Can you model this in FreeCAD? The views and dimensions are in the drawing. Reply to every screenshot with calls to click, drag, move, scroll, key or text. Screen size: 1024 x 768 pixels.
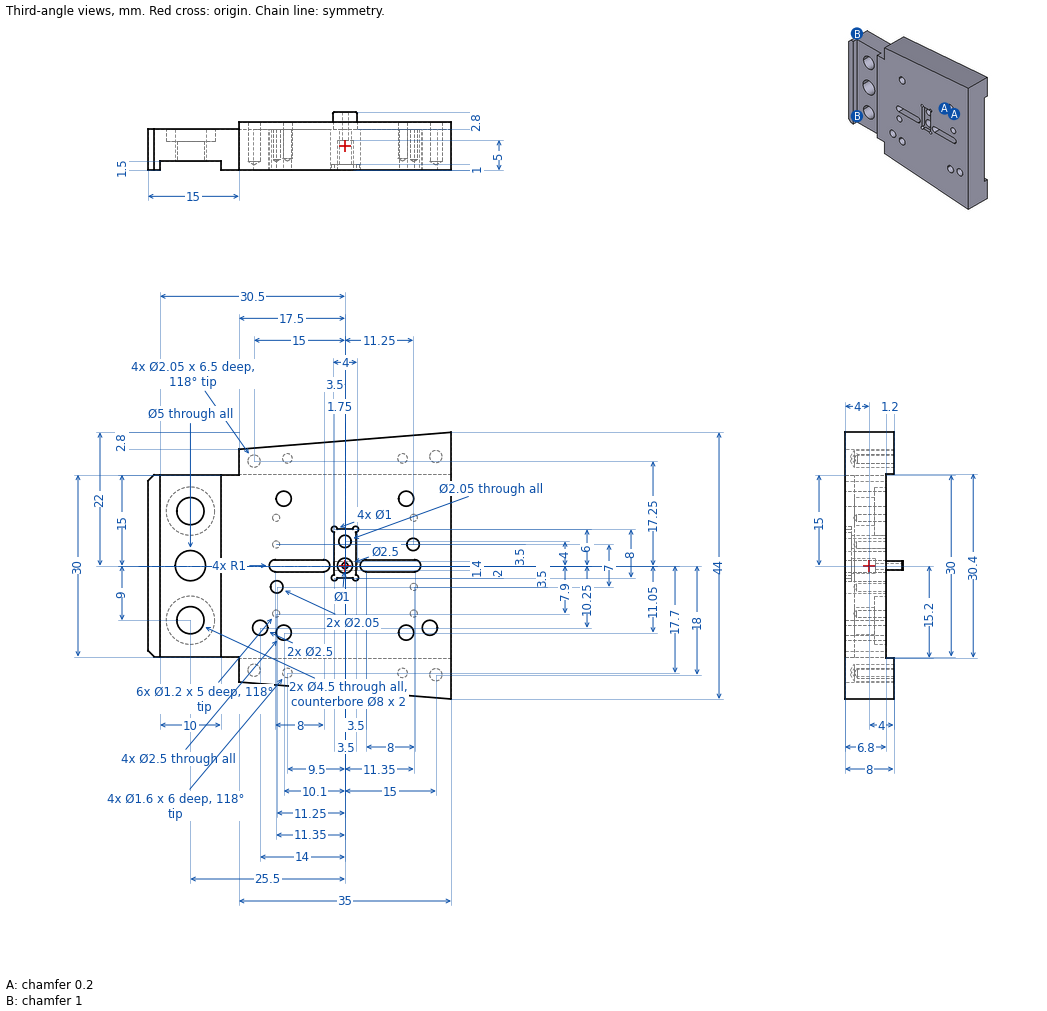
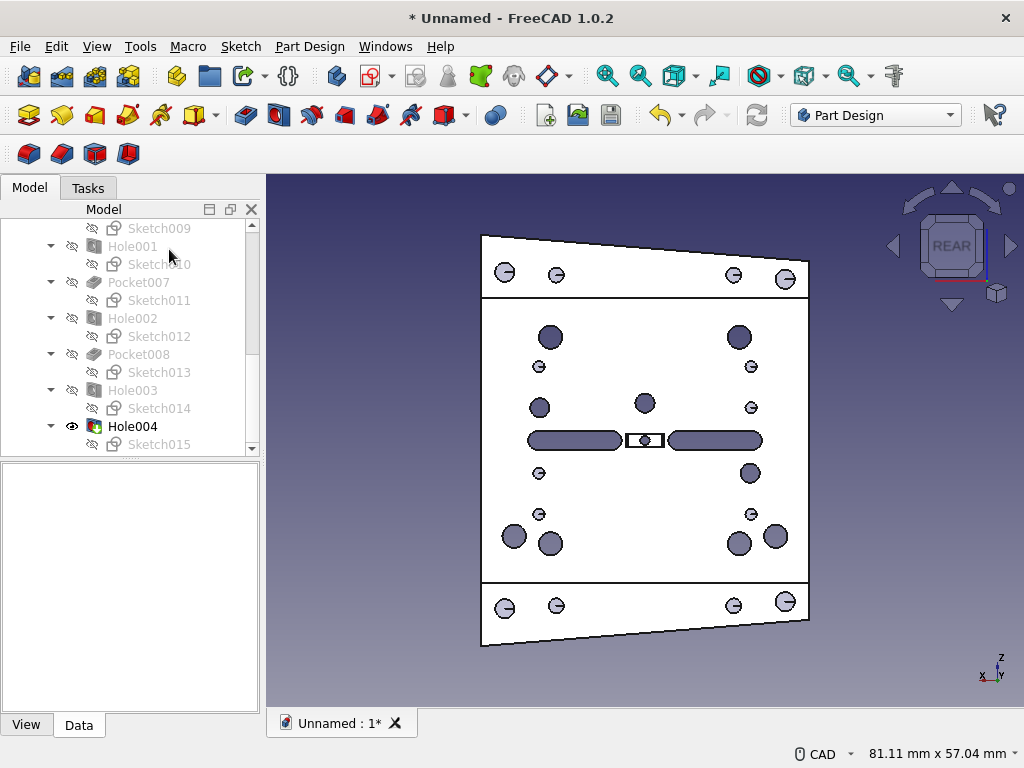
key(6)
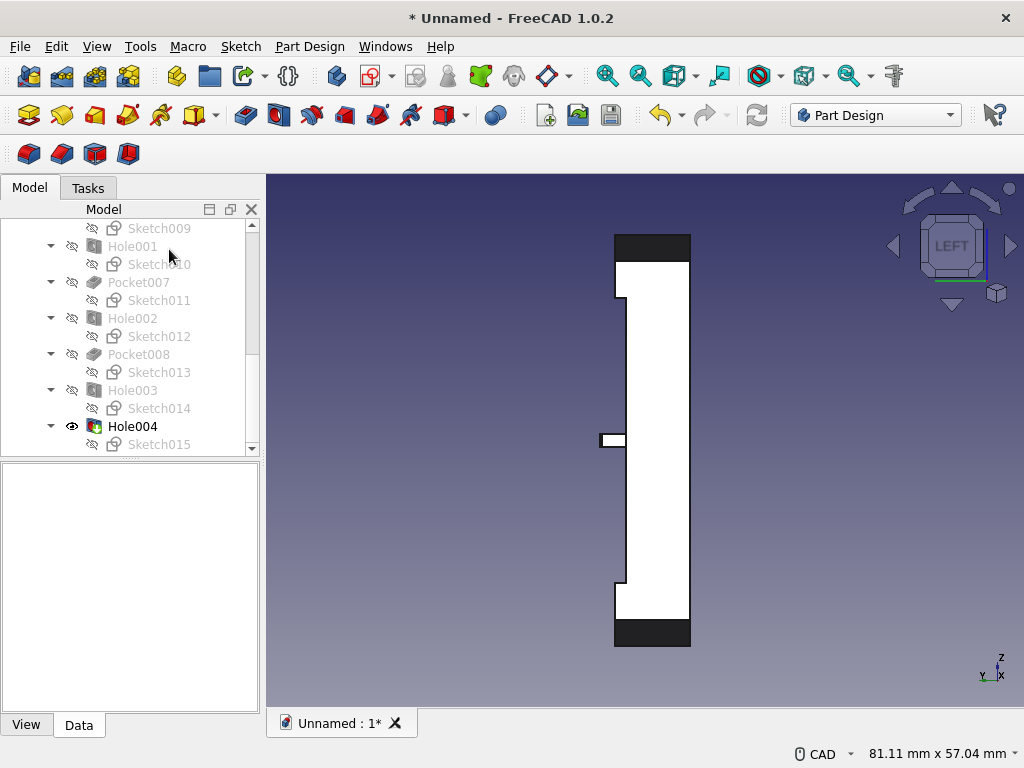
click(663, 440)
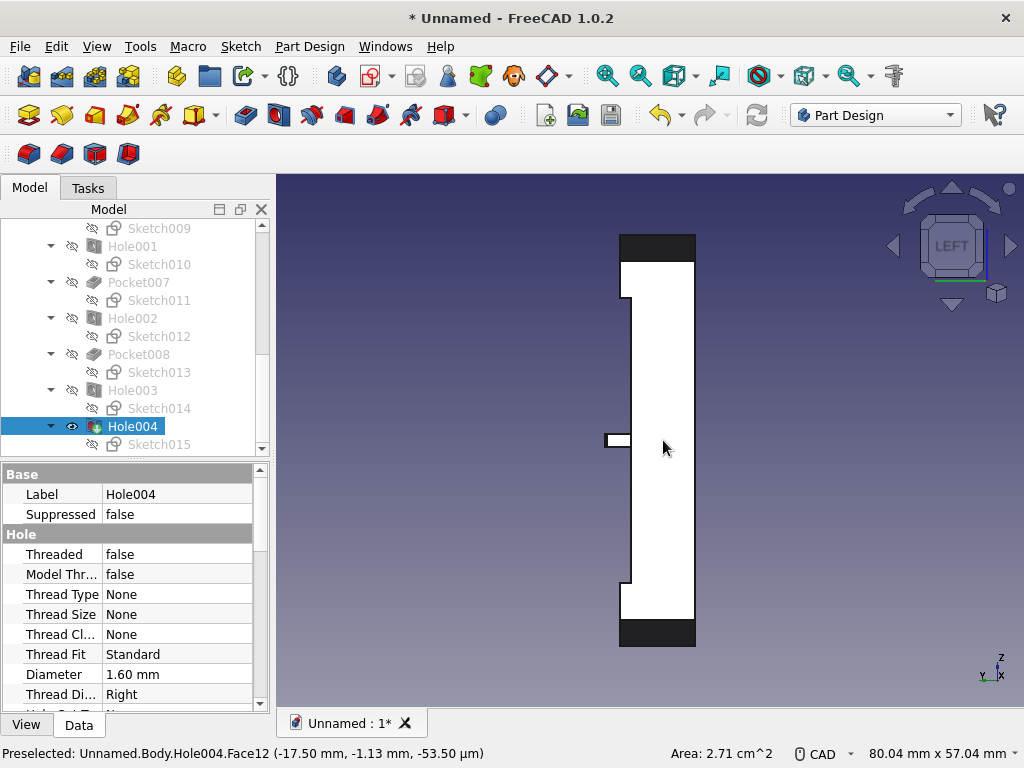
click(370, 76)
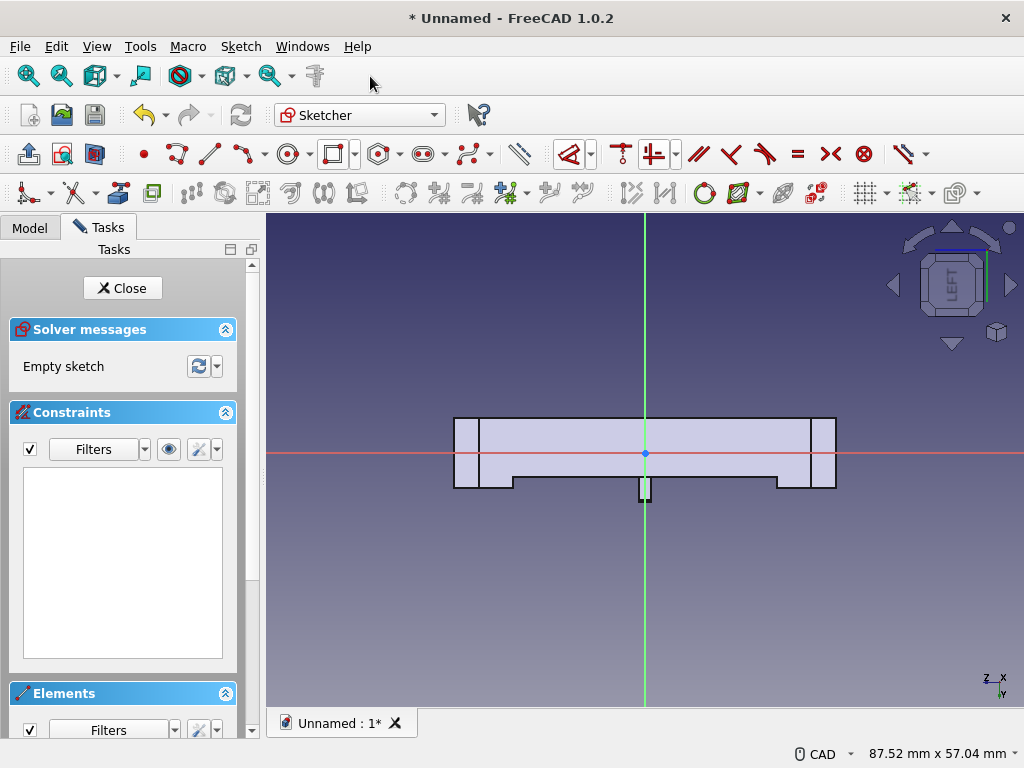
scroll(784, 423, up, 2)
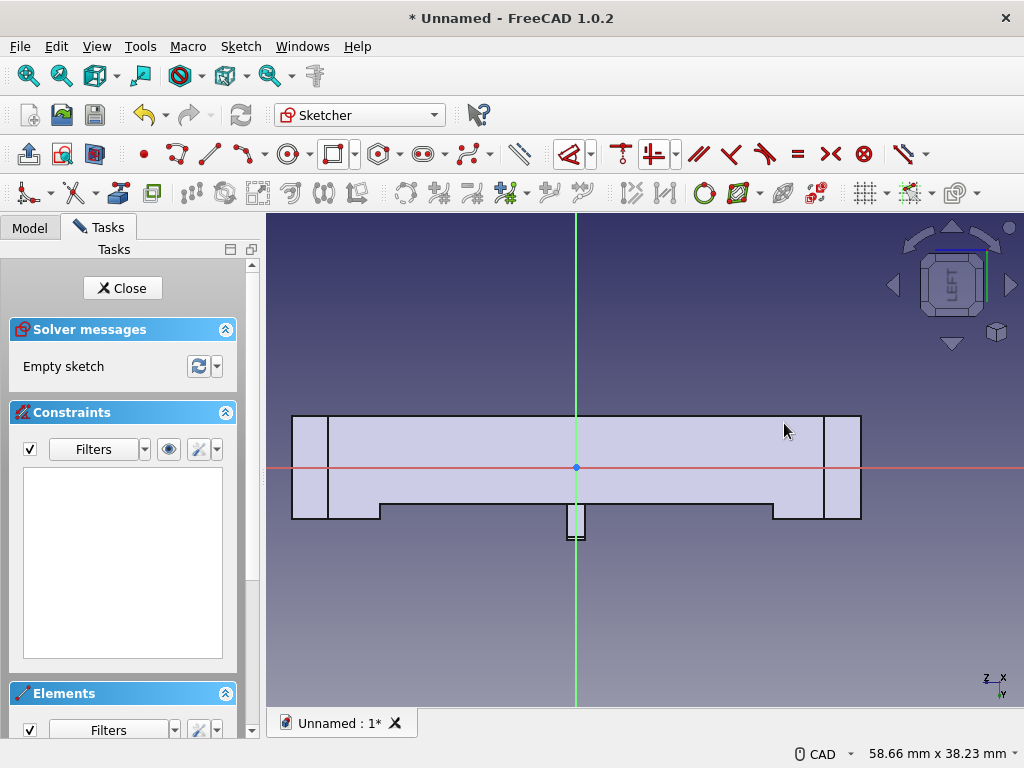
click(332, 154)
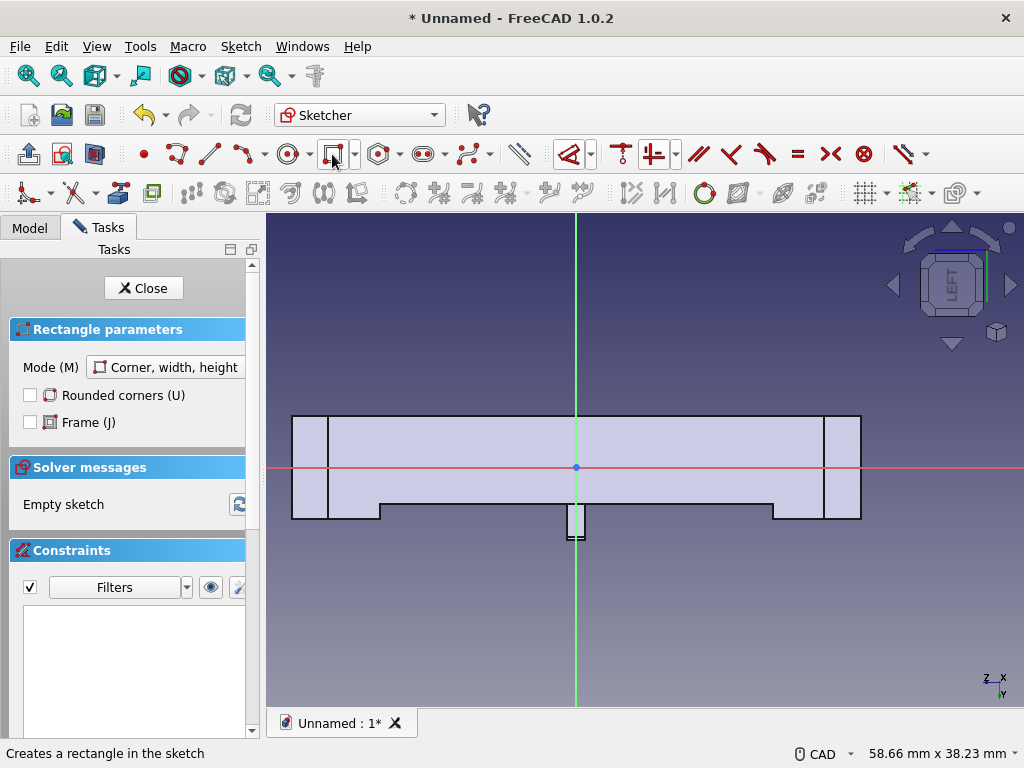
click(382, 416)
move(770, 504)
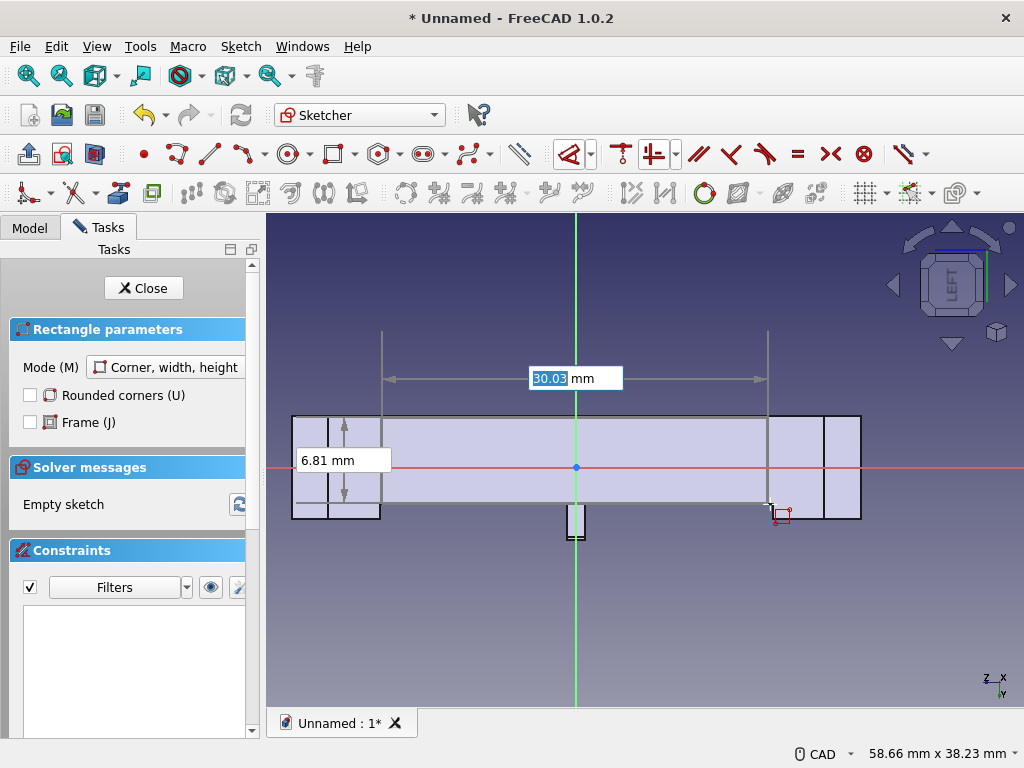
text(30)
key(Tab)
text(6.8)
key(Return)
key(Escape)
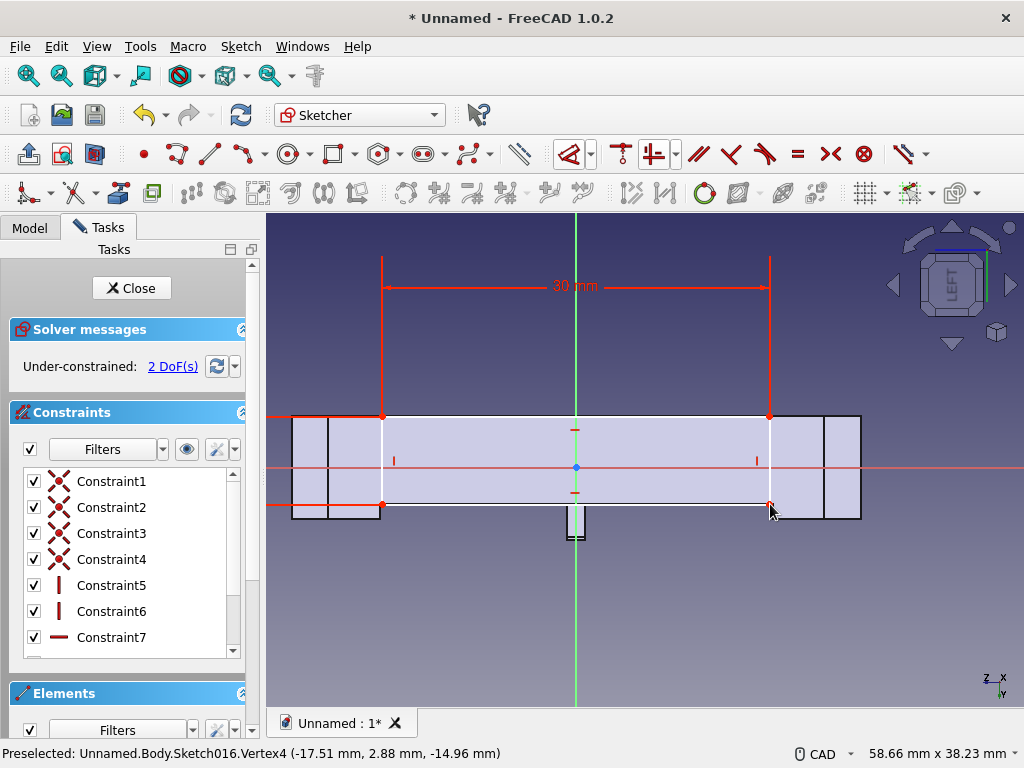
click(382, 417)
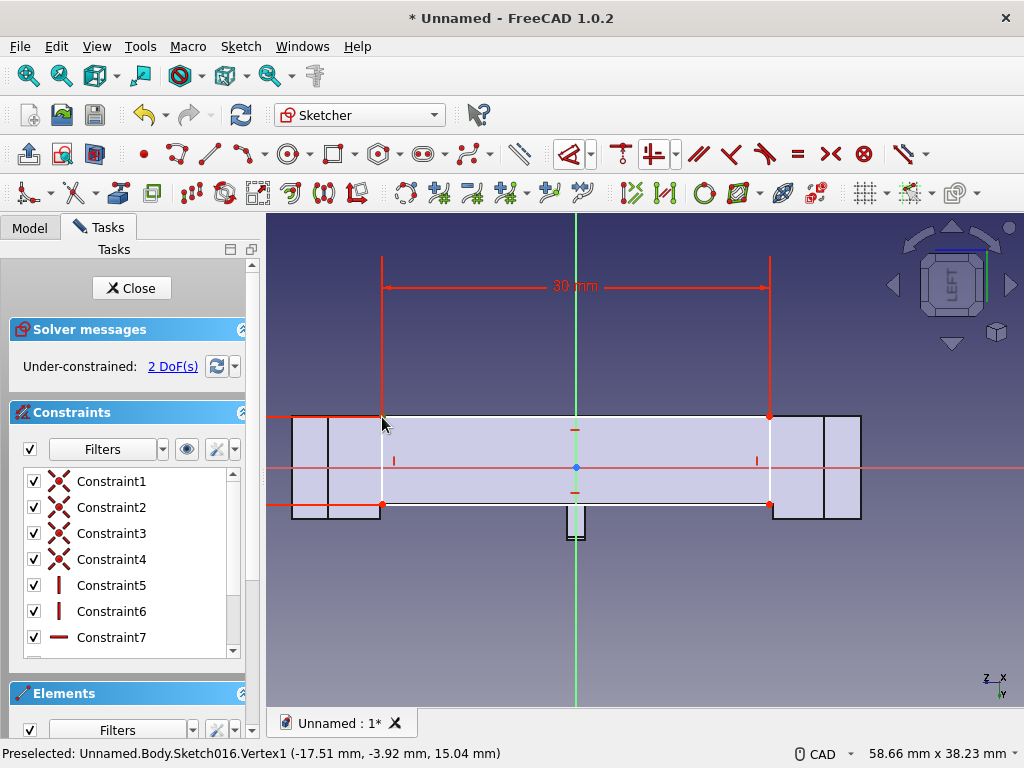
key(i)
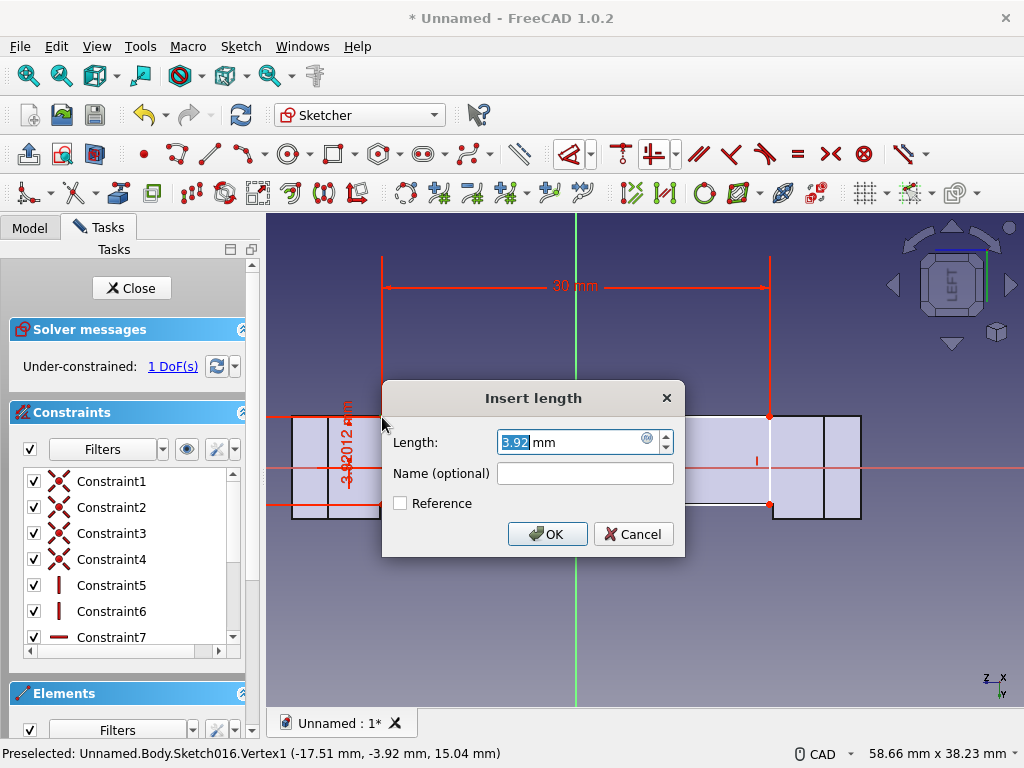
text(4)
key(Return)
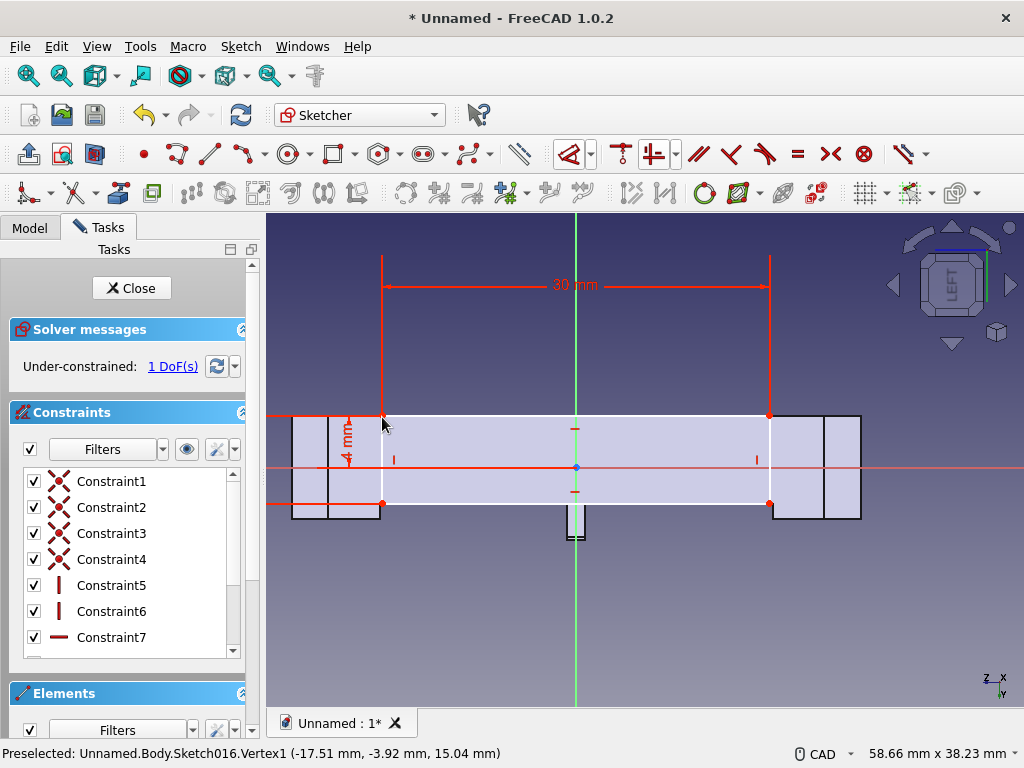
click(382, 416)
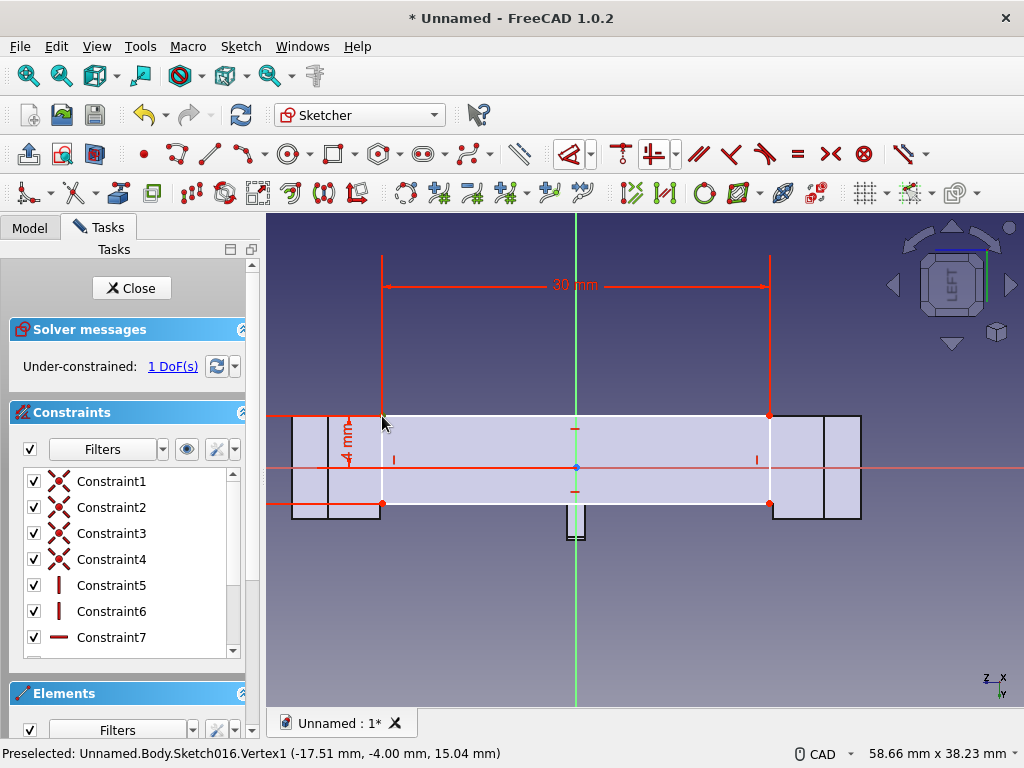
click(590, 154)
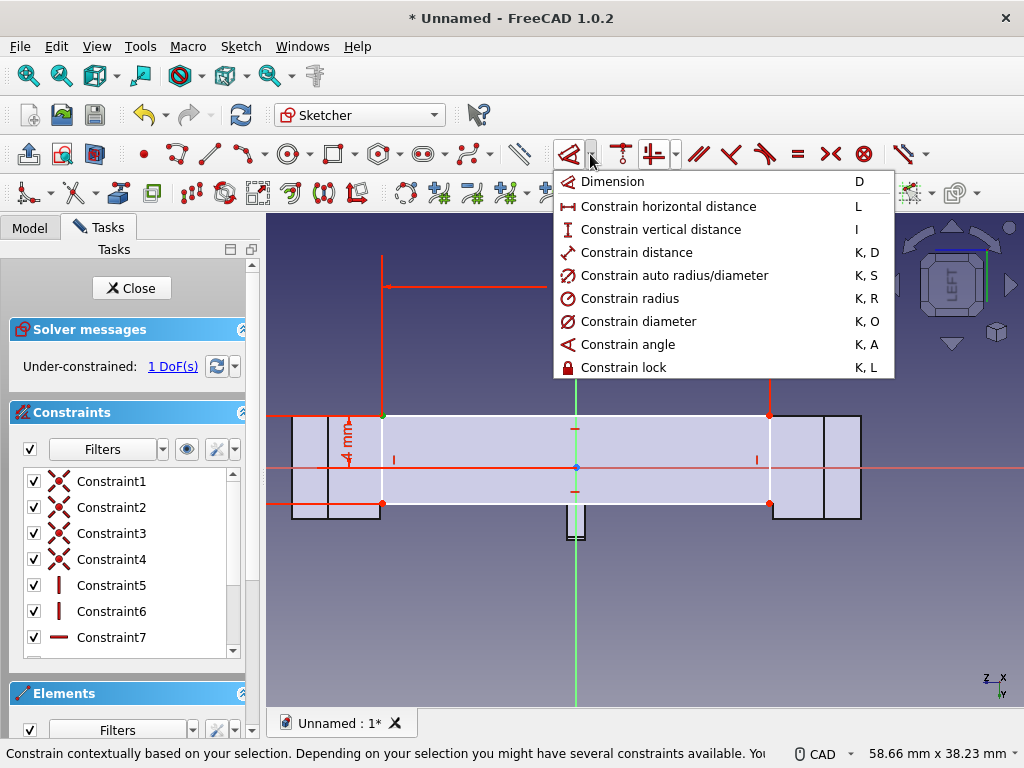
click(724, 206)